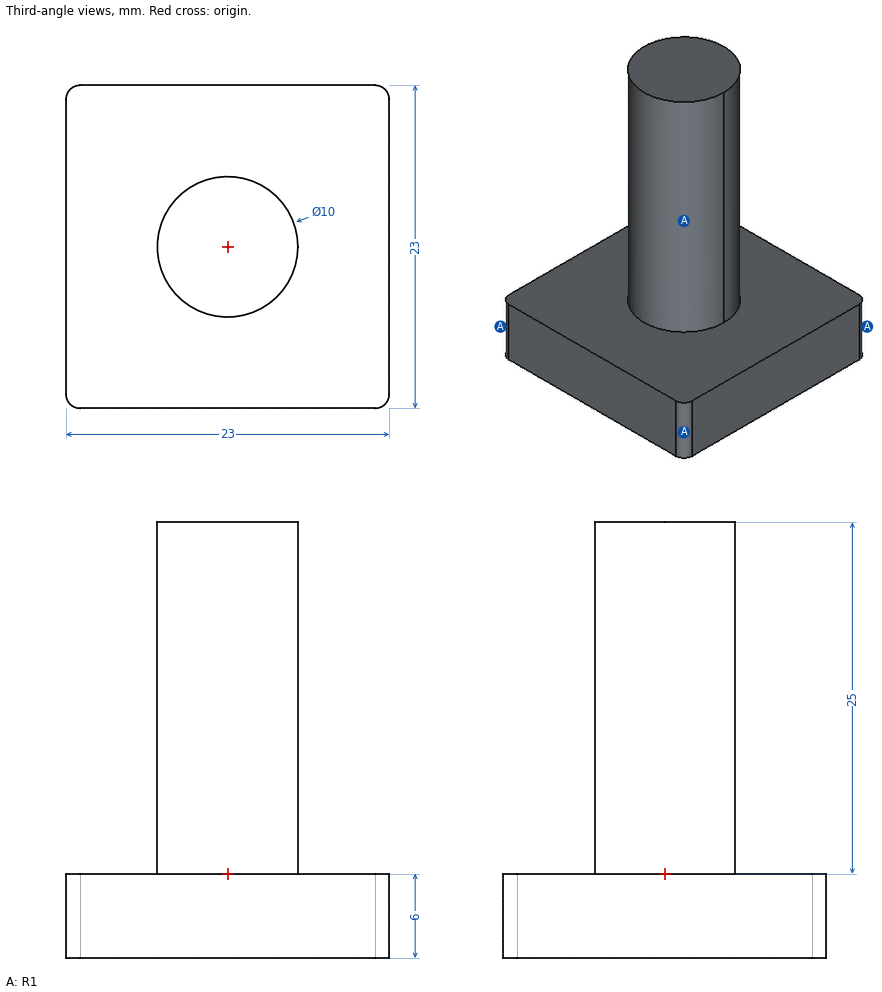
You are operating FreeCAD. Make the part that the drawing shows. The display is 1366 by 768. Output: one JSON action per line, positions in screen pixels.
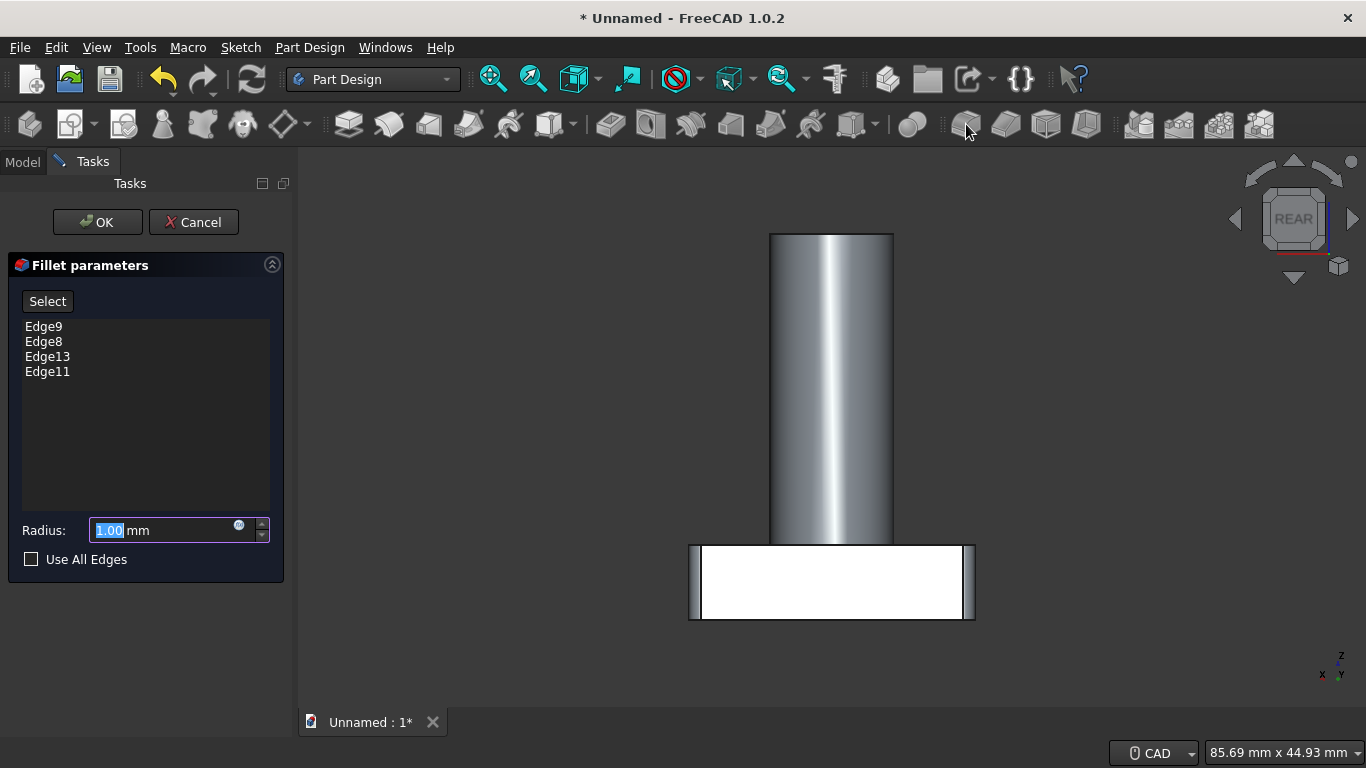
{"action": "type", "text": "1"}
{"action": "key", "text": "Tab"}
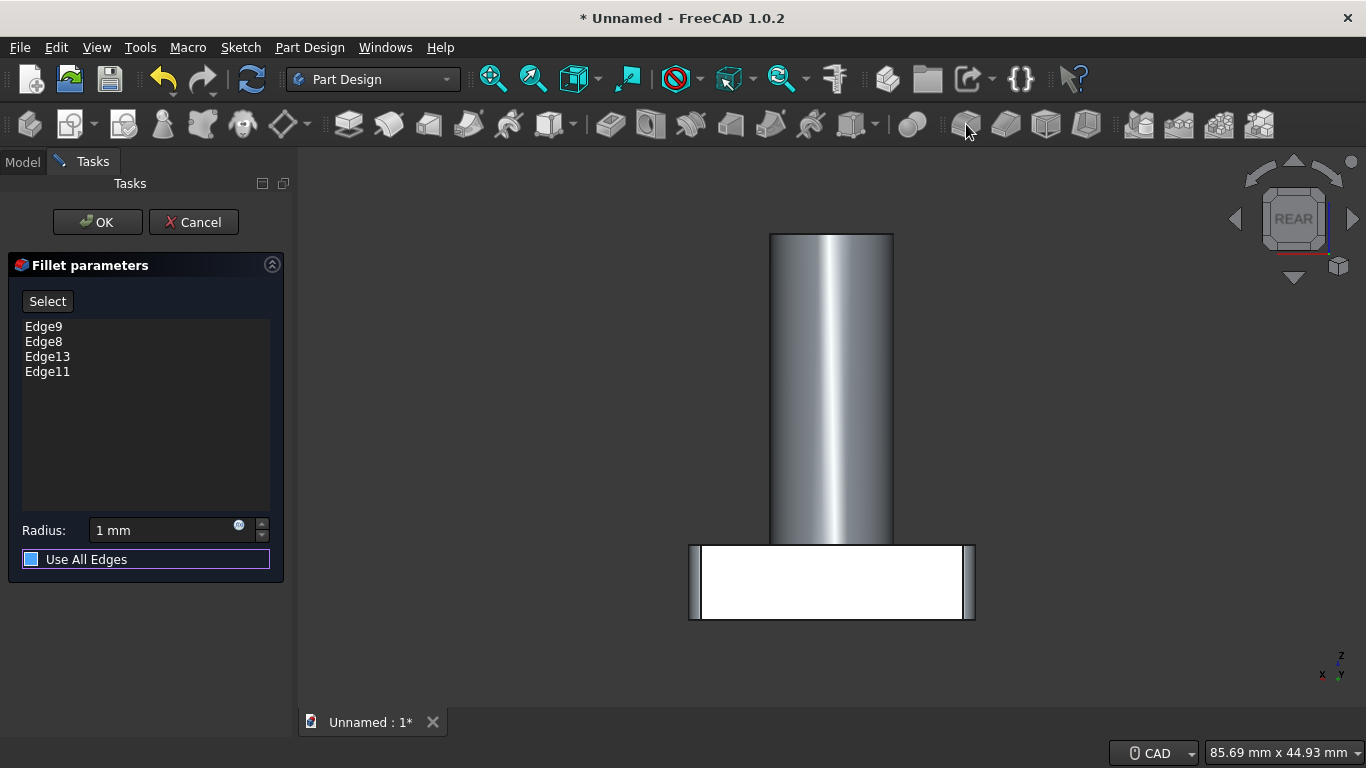
{"action": "left_click", "coordinate": [98, 222]}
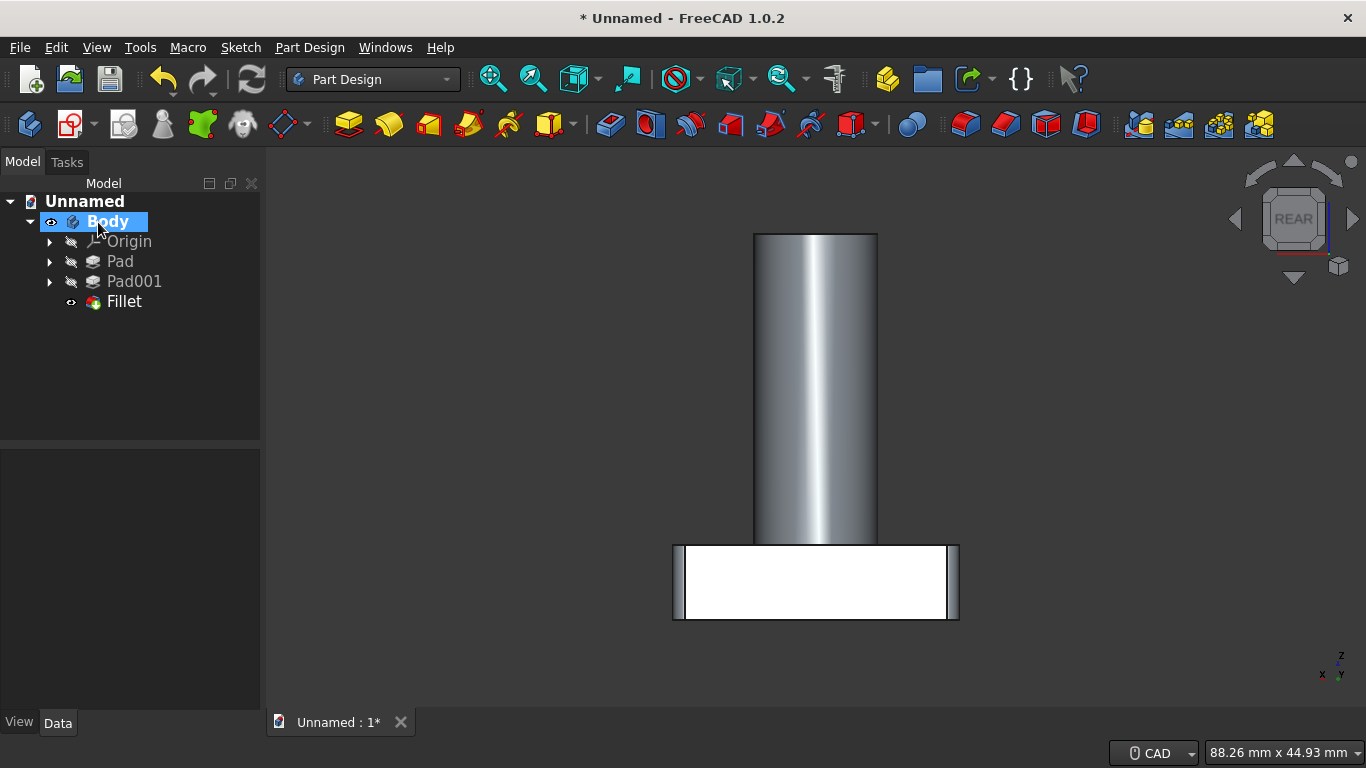
{"action": "key", "text": "0"}